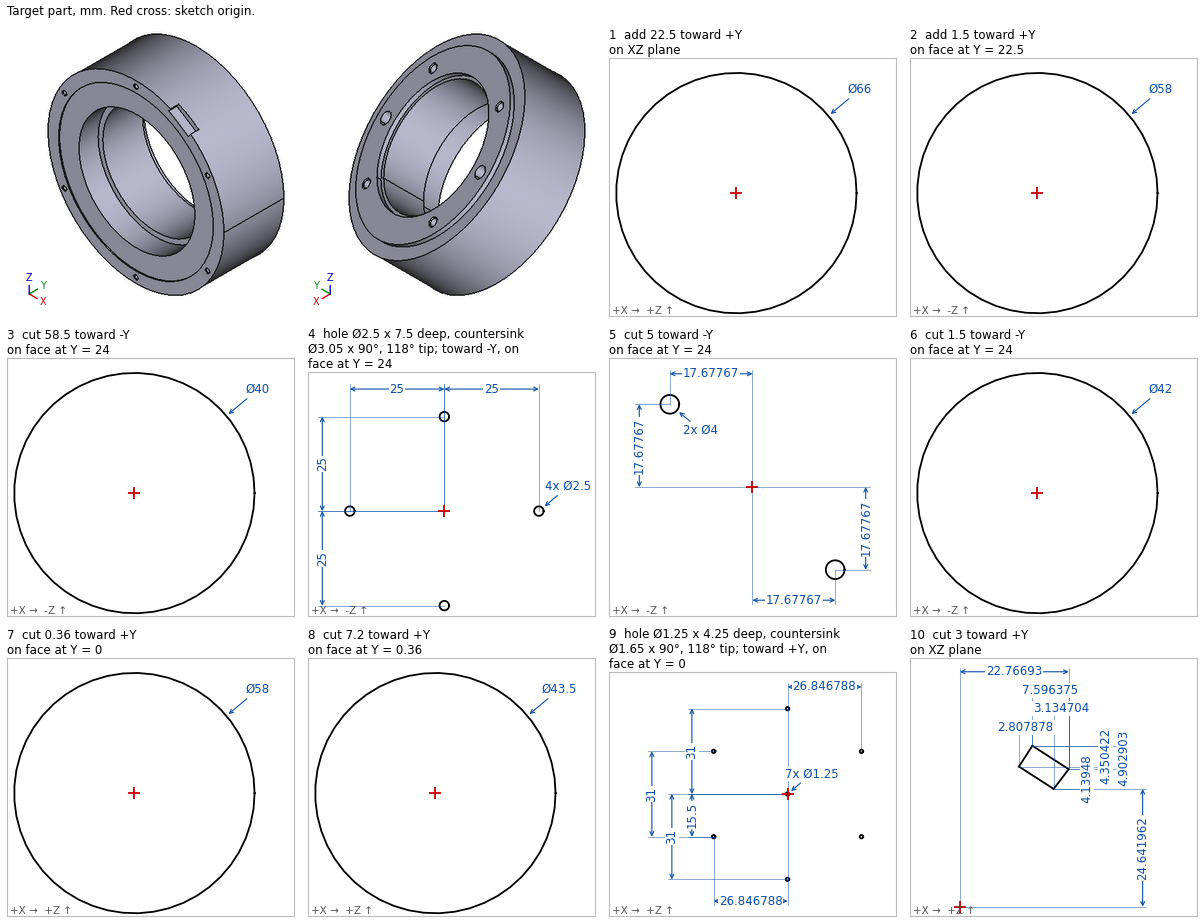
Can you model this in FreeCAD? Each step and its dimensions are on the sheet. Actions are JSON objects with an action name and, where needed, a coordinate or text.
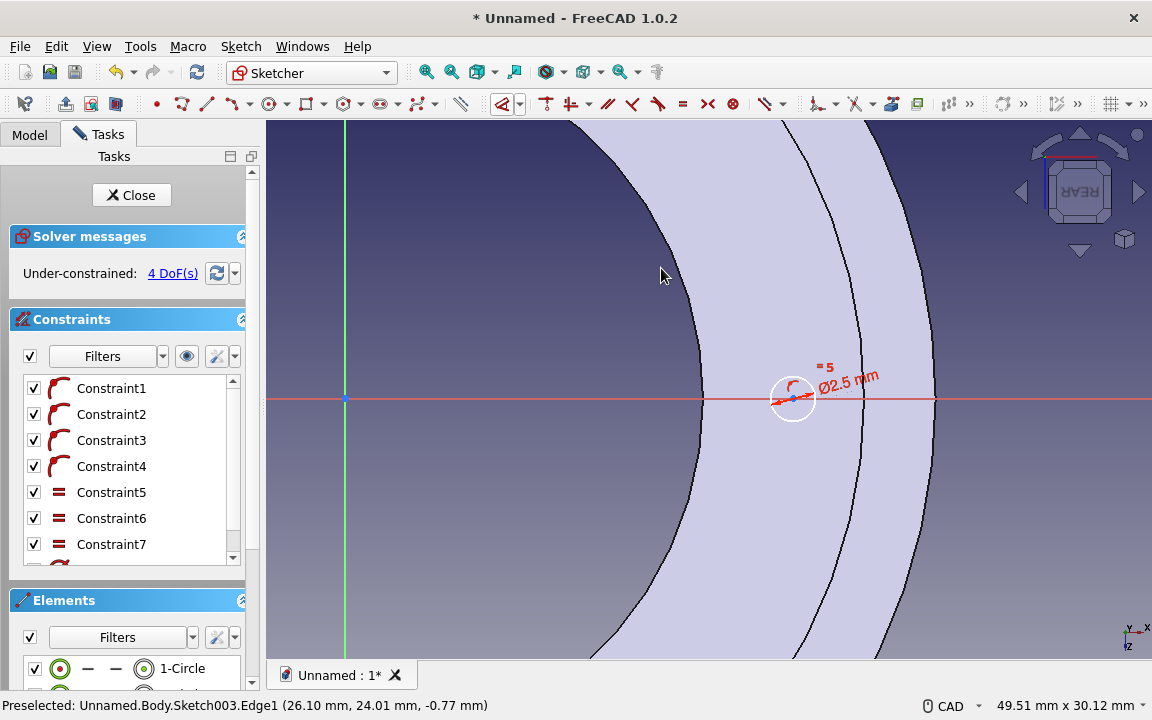
{"action": "left_click", "coordinate": [793, 399]}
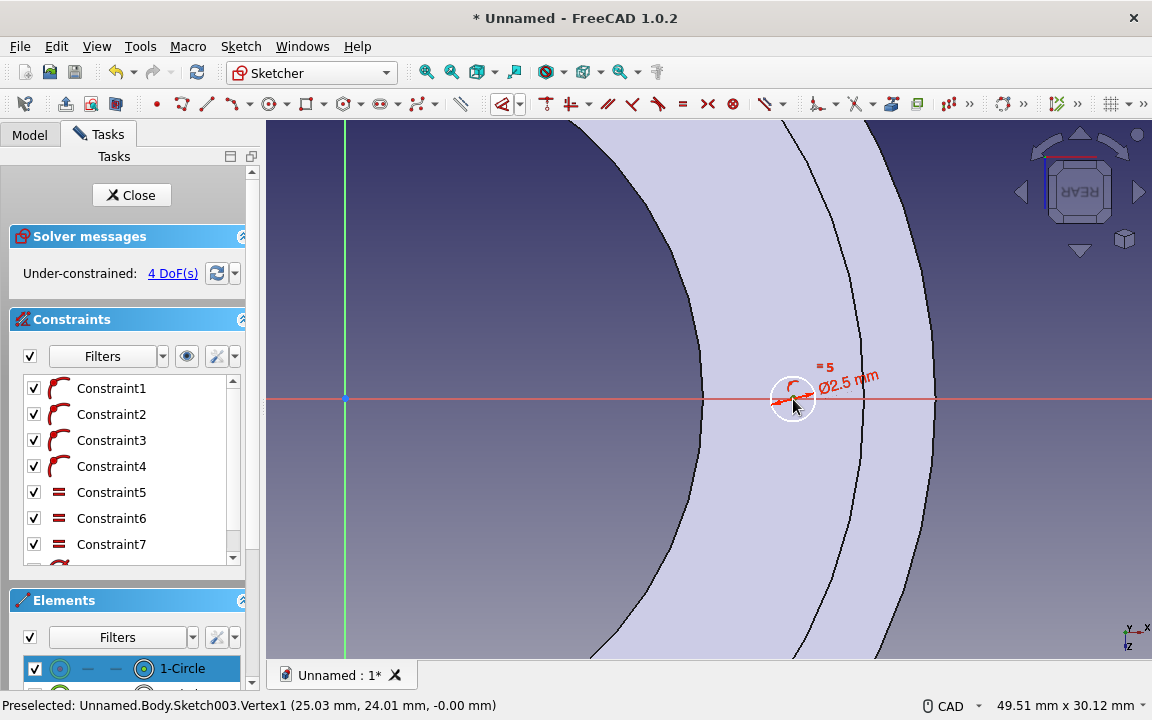
{"action": "left_click", "coordinate": [520, 104]}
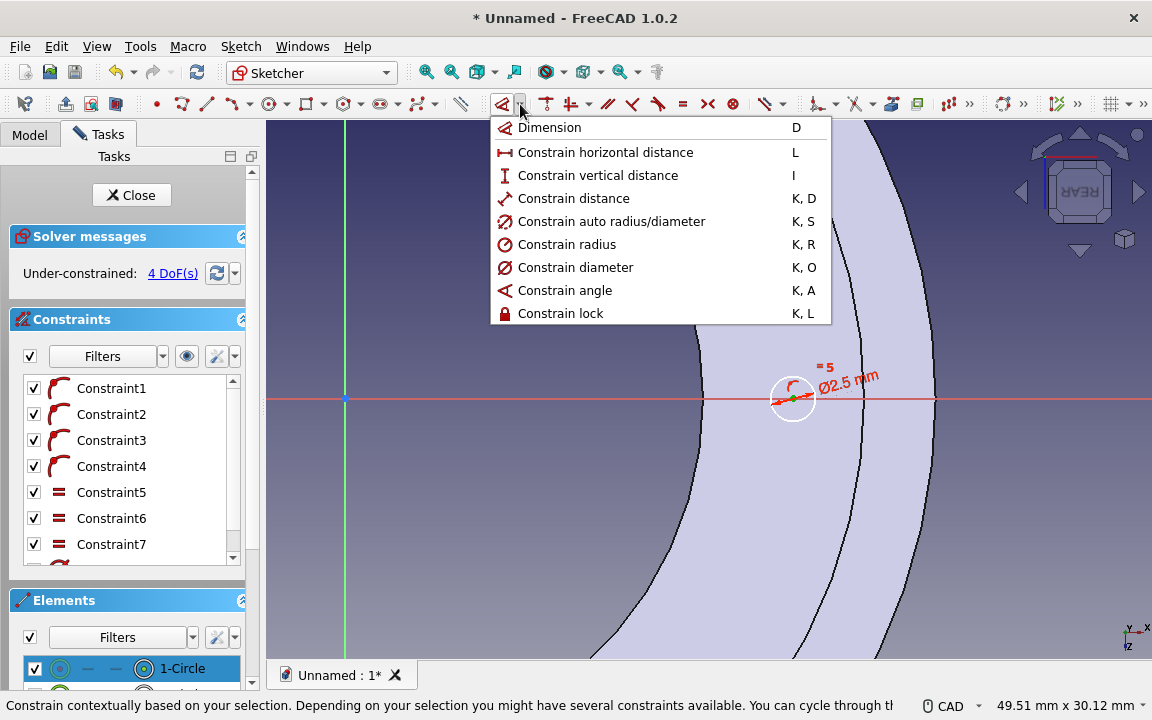
{"action": "left_click", "coordinate": [661, 152]}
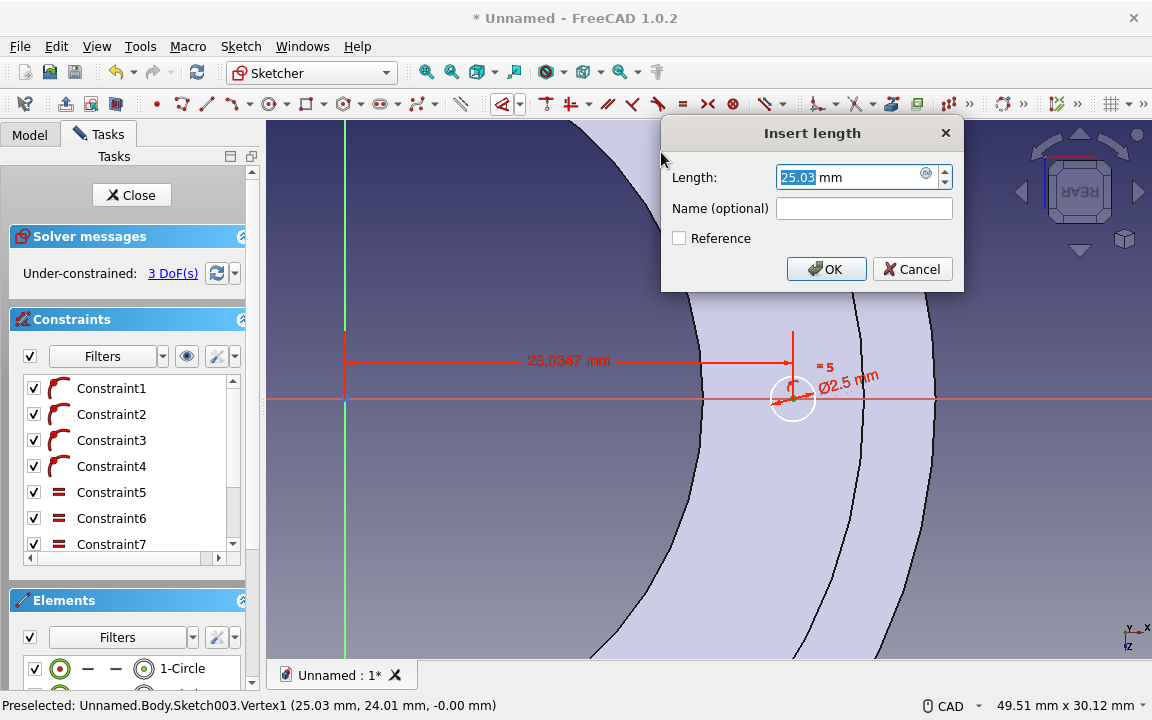
{"action": "type", "text": "25"}
{"action": "key", "text": "Return"}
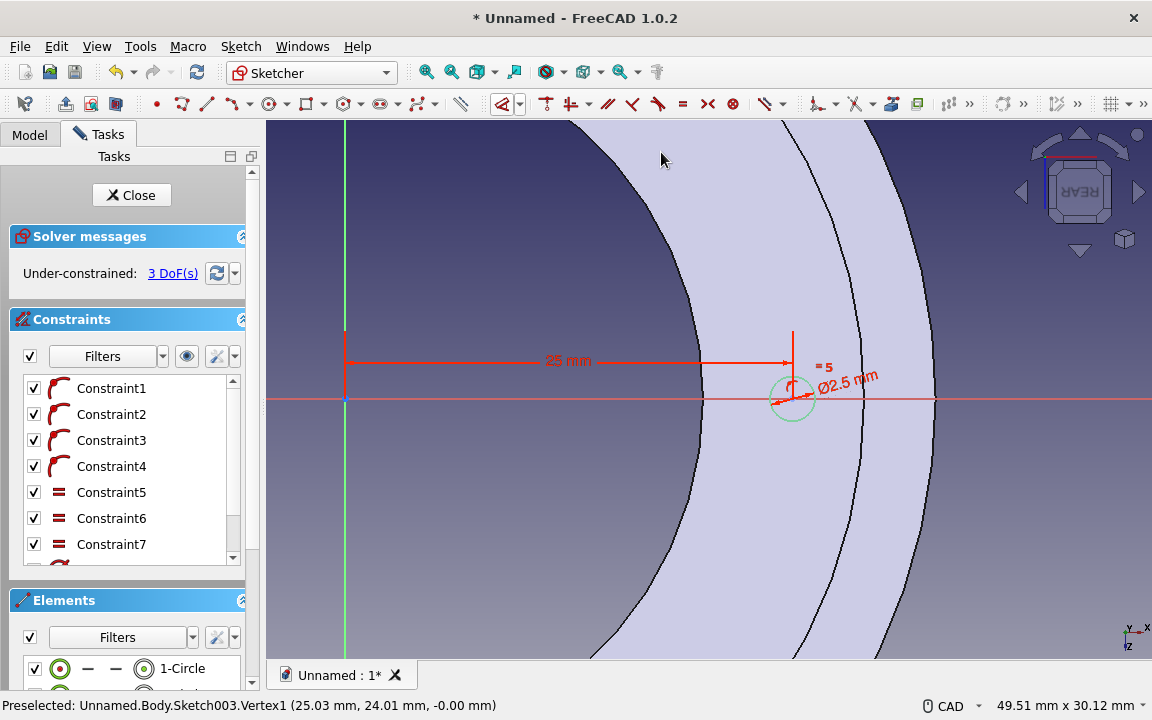
{"action": "scroll", "coordinate": [812, 384], "scroll_direction": "down", "scroll_amount": 5}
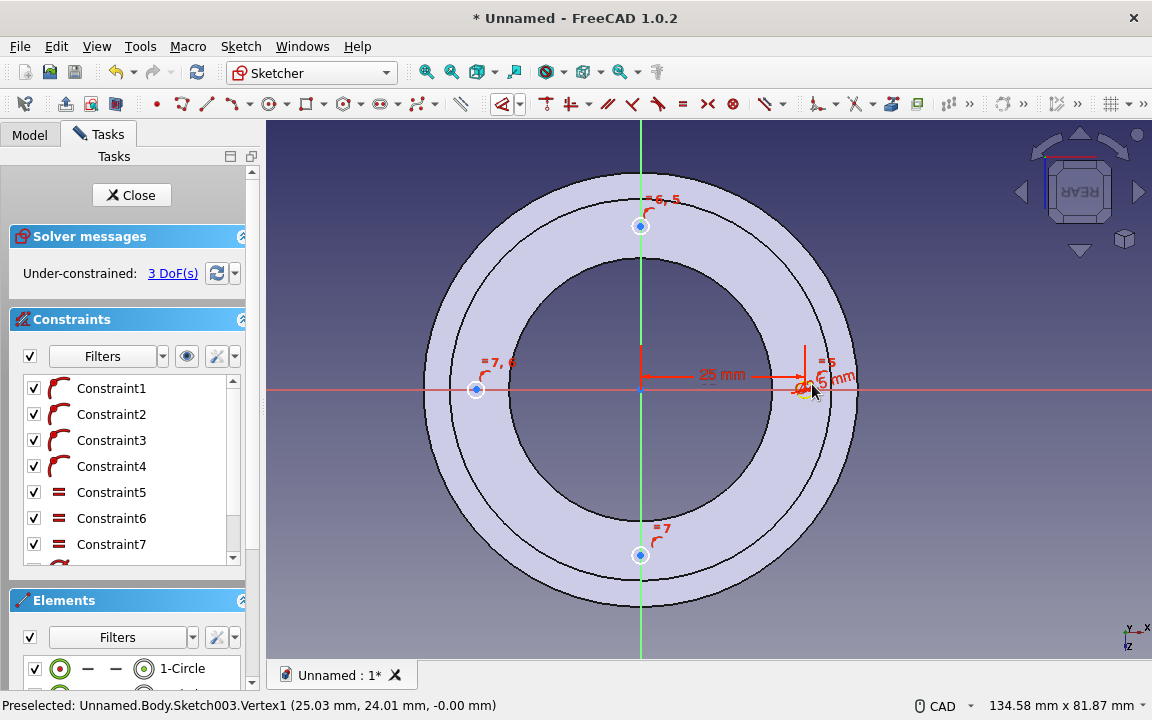
{"action": "left_click", "coordinate": [641, 226]}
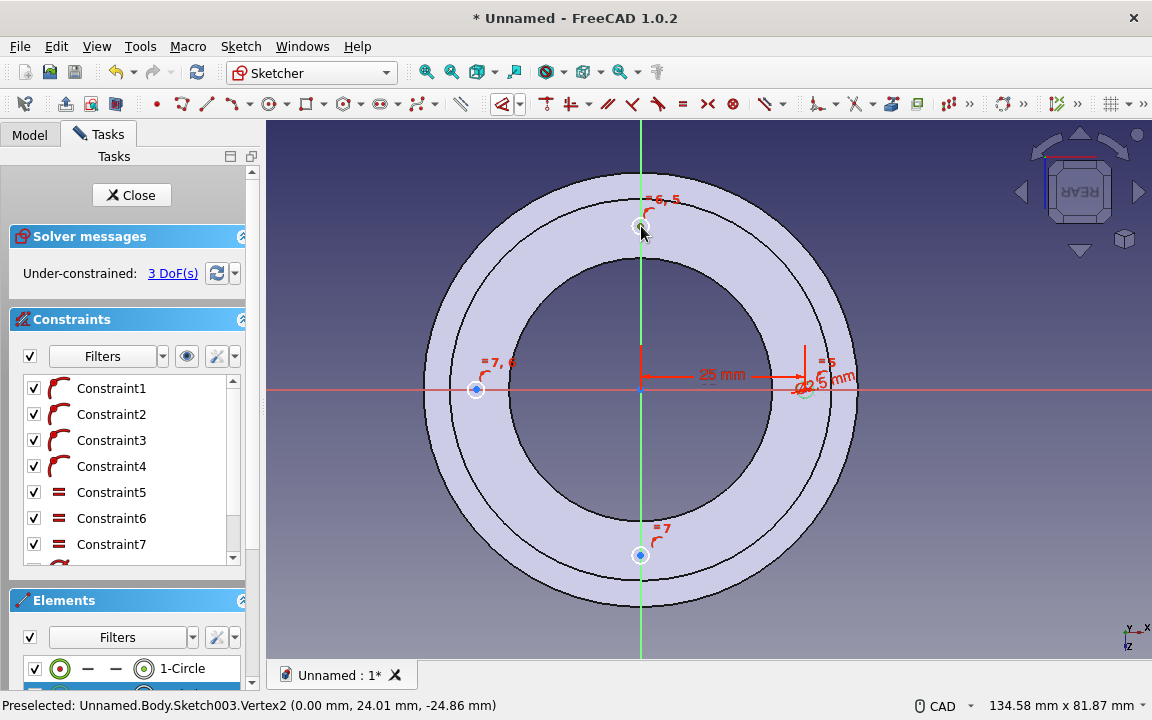
{"action": "left_click", "coordinate": [520, 104]}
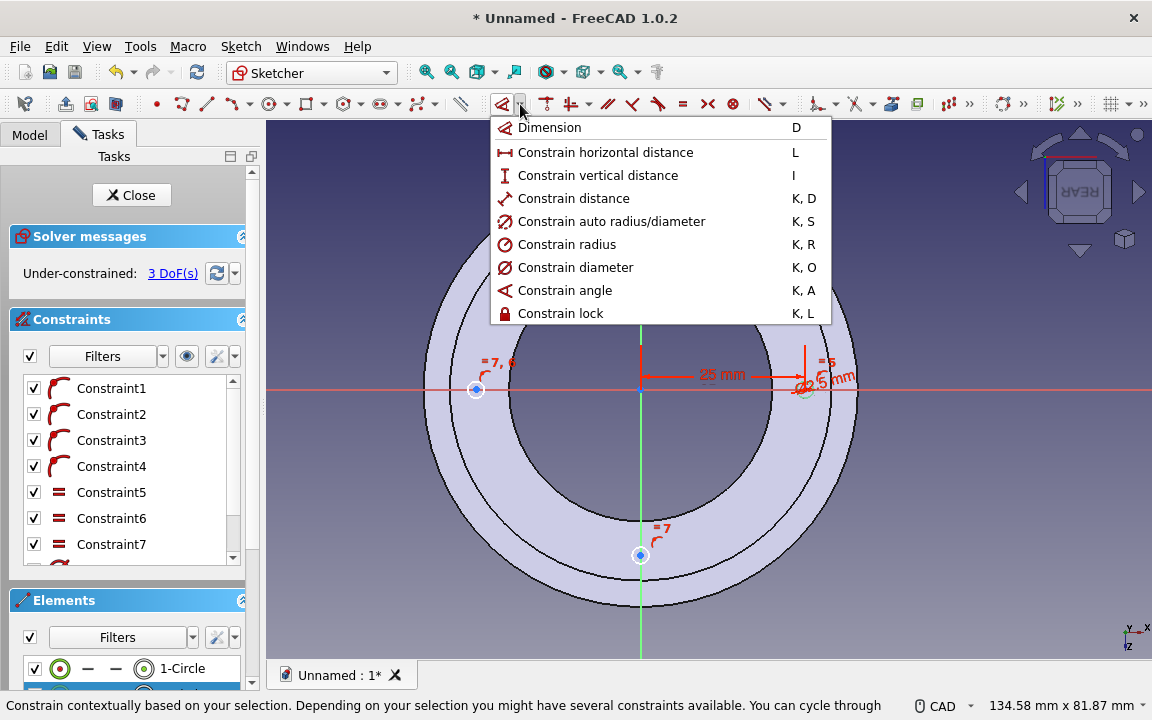
{"action": "left_click", "coordinate": [661, 176]}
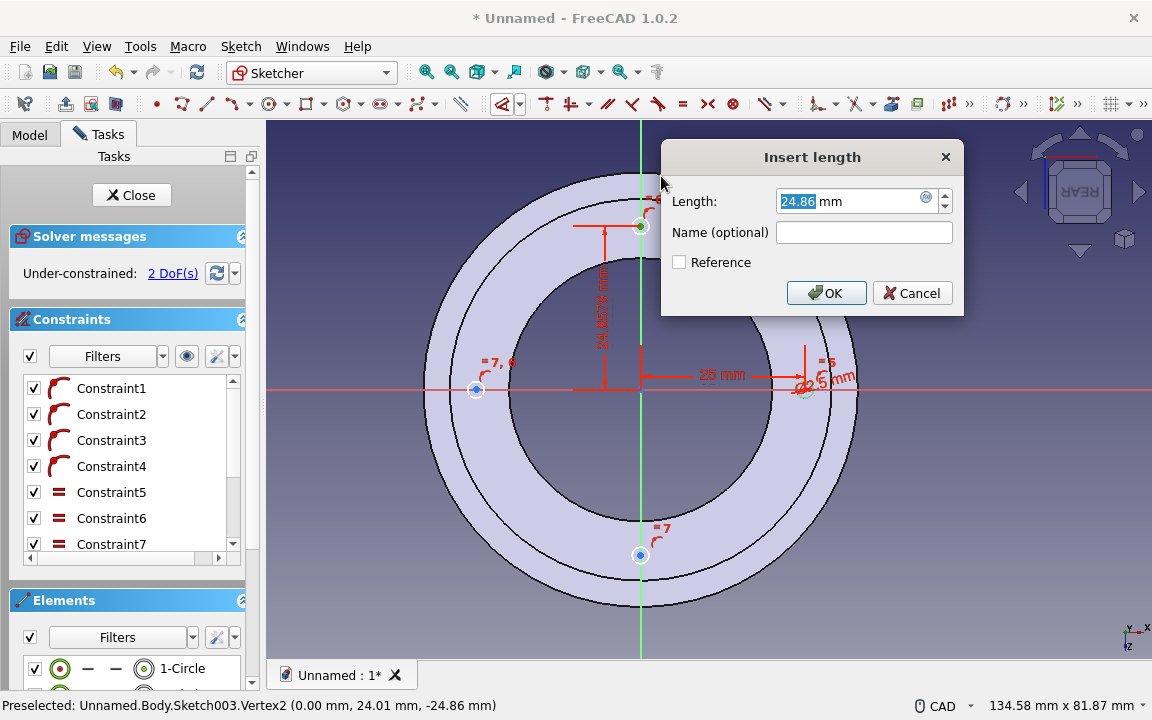
{"action": "type", "text": "25"}
{"action": "key", "text": "Return"}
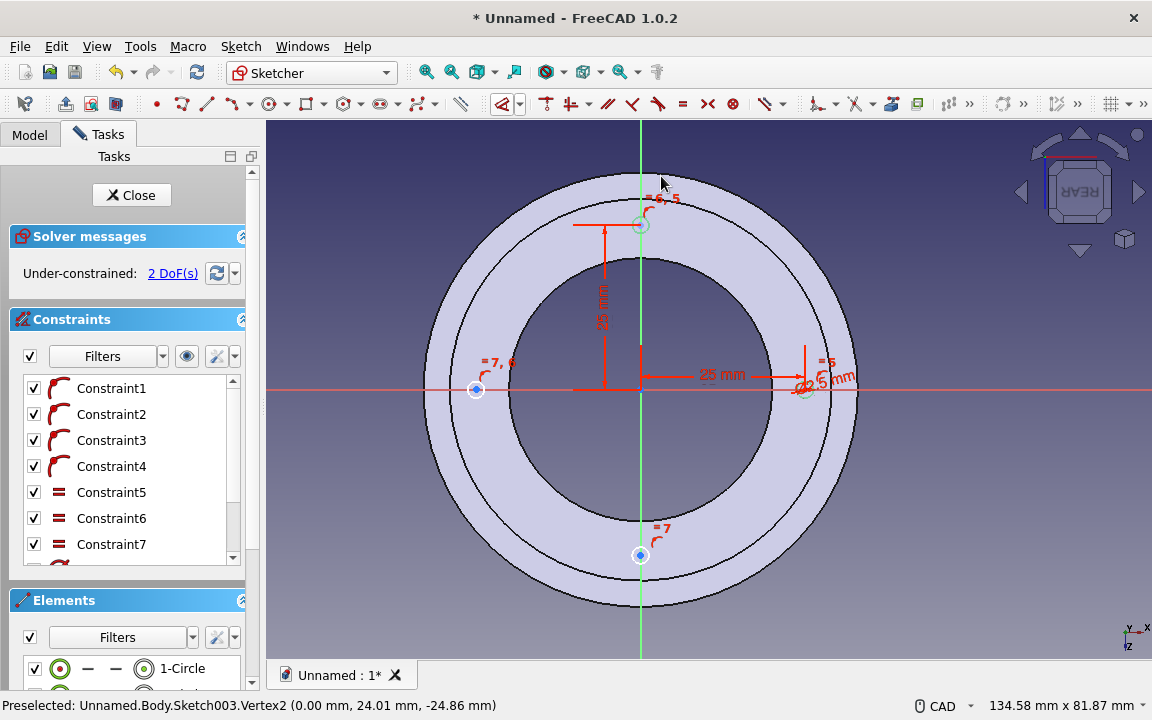
{"action": "left_click", "coordinate": [476, 390]}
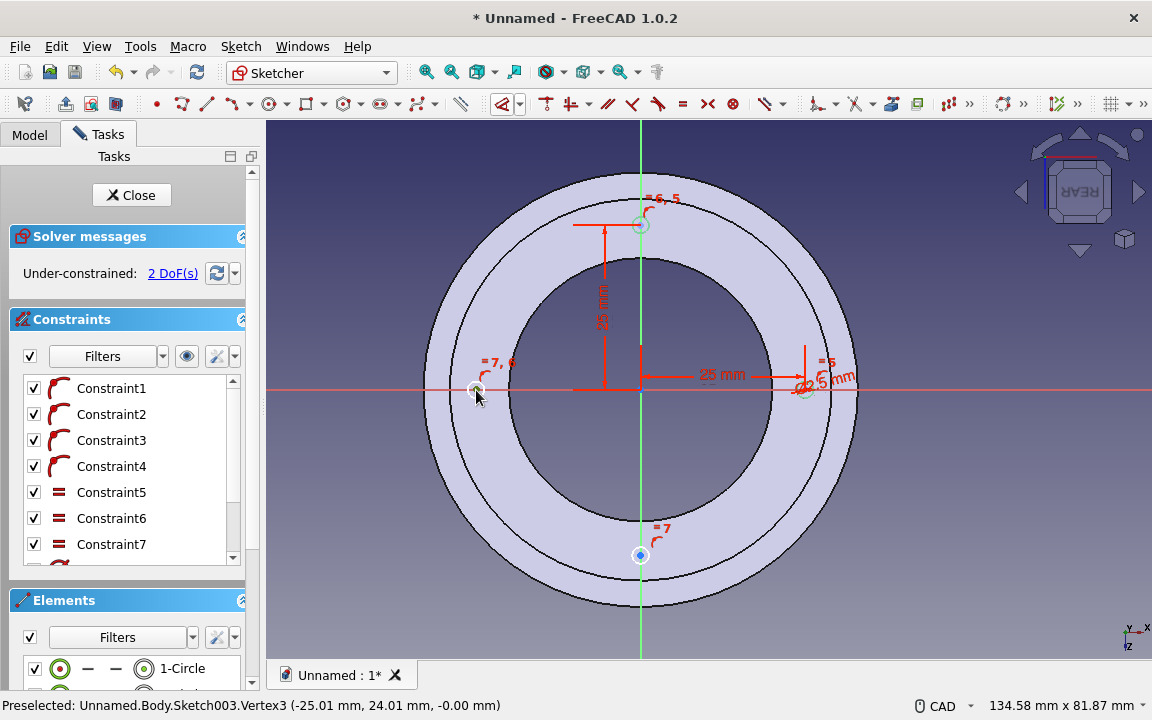
{"action": "key", "text": "l"}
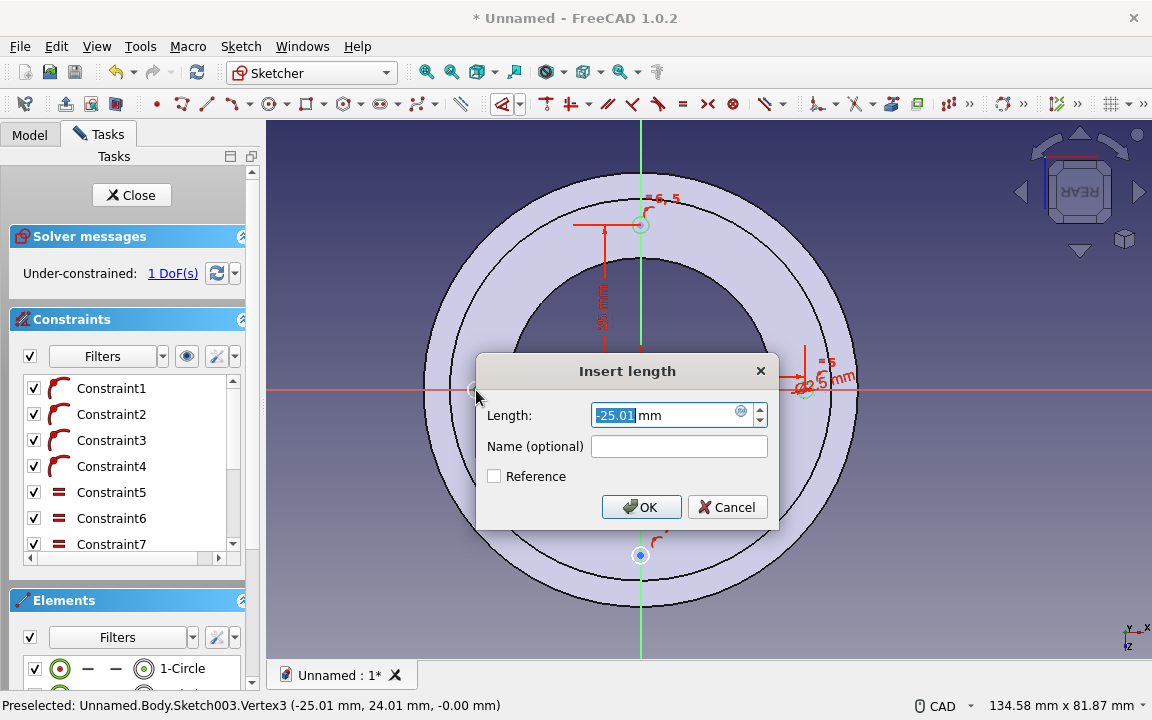
{"action": "type", "text": "-25"}
{"action": "key", "text": "Return"}